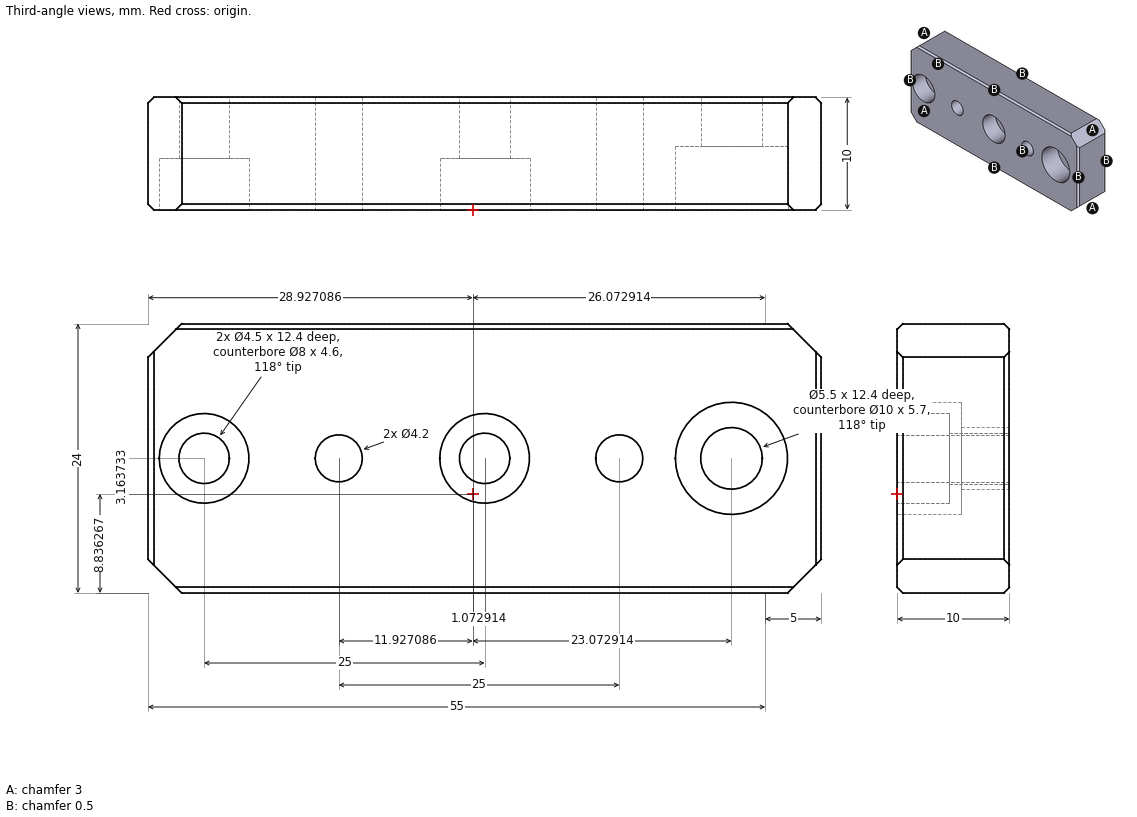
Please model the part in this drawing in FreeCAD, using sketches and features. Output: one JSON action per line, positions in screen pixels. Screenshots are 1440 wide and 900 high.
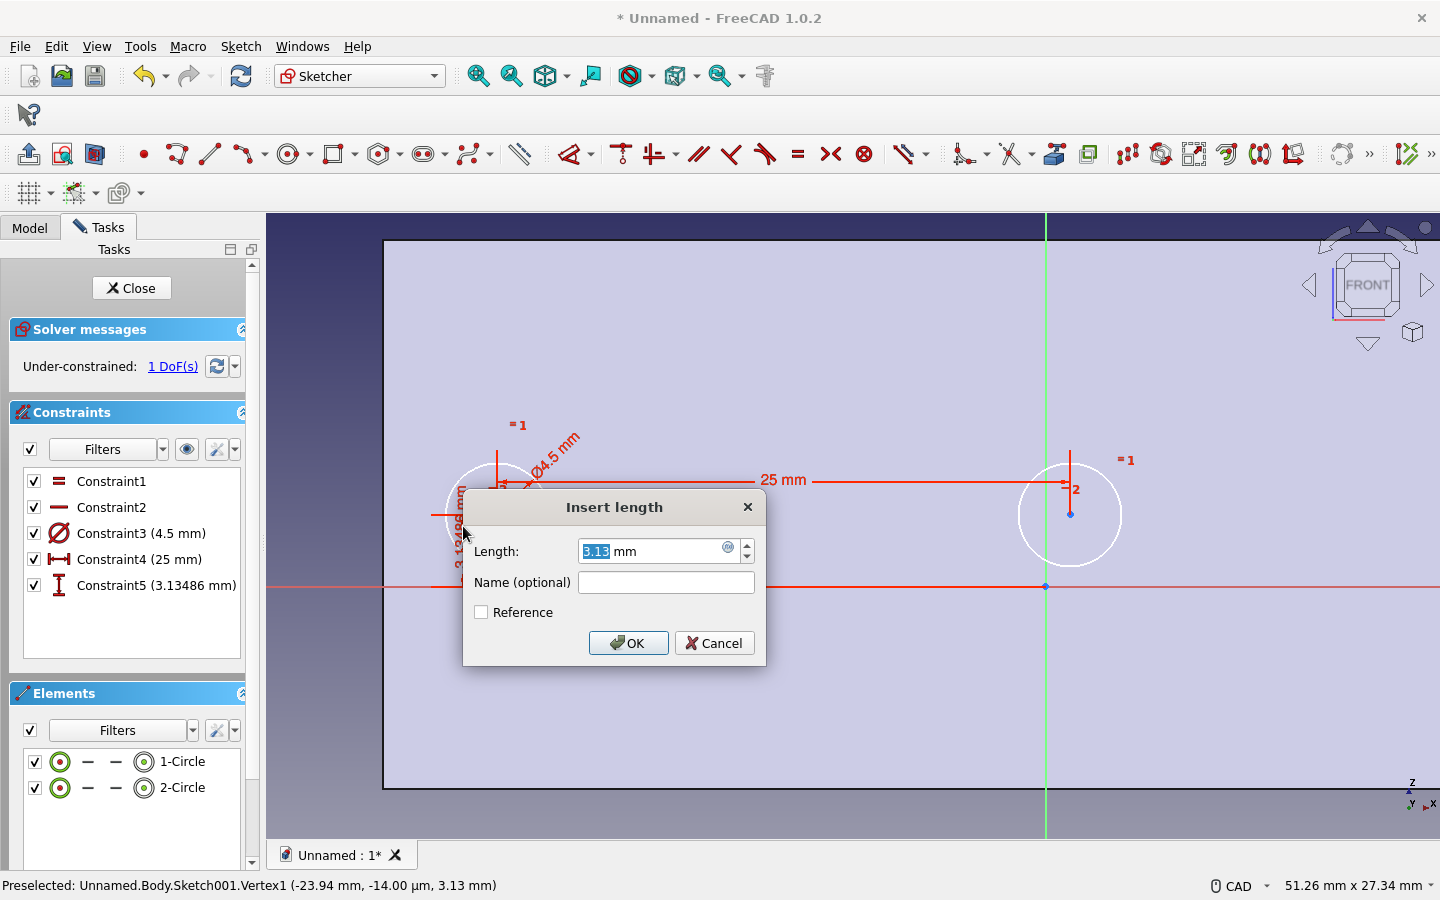
{"action": "type", "text": "3.163733"}
{"action": "key", "text": "Return"}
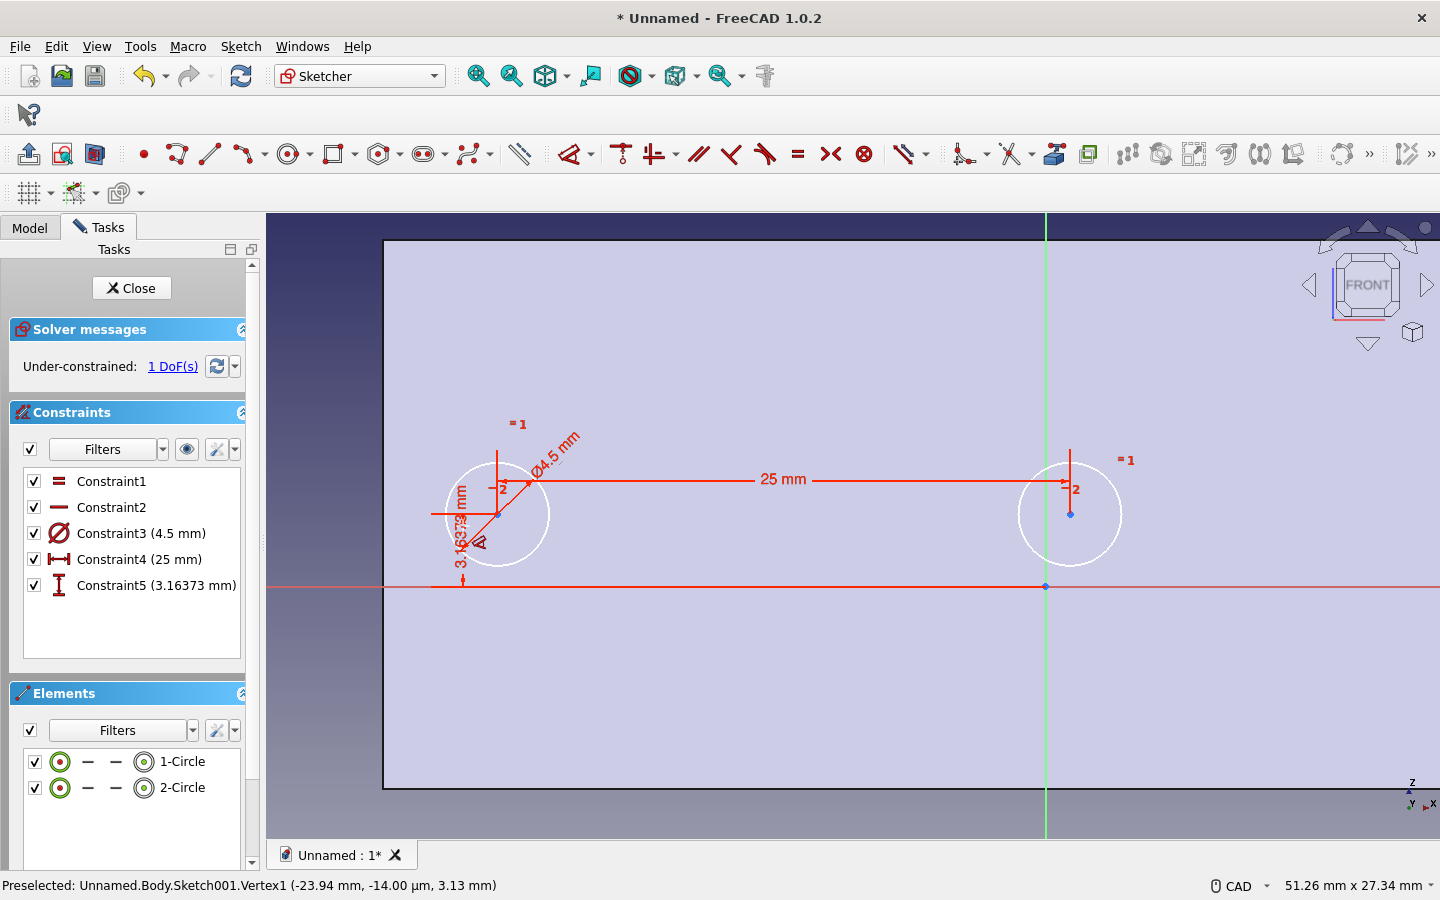
{"action": "scroll", "coordinate": [1070, 514], "scroll_direction": "up", "scroll_amount": 3}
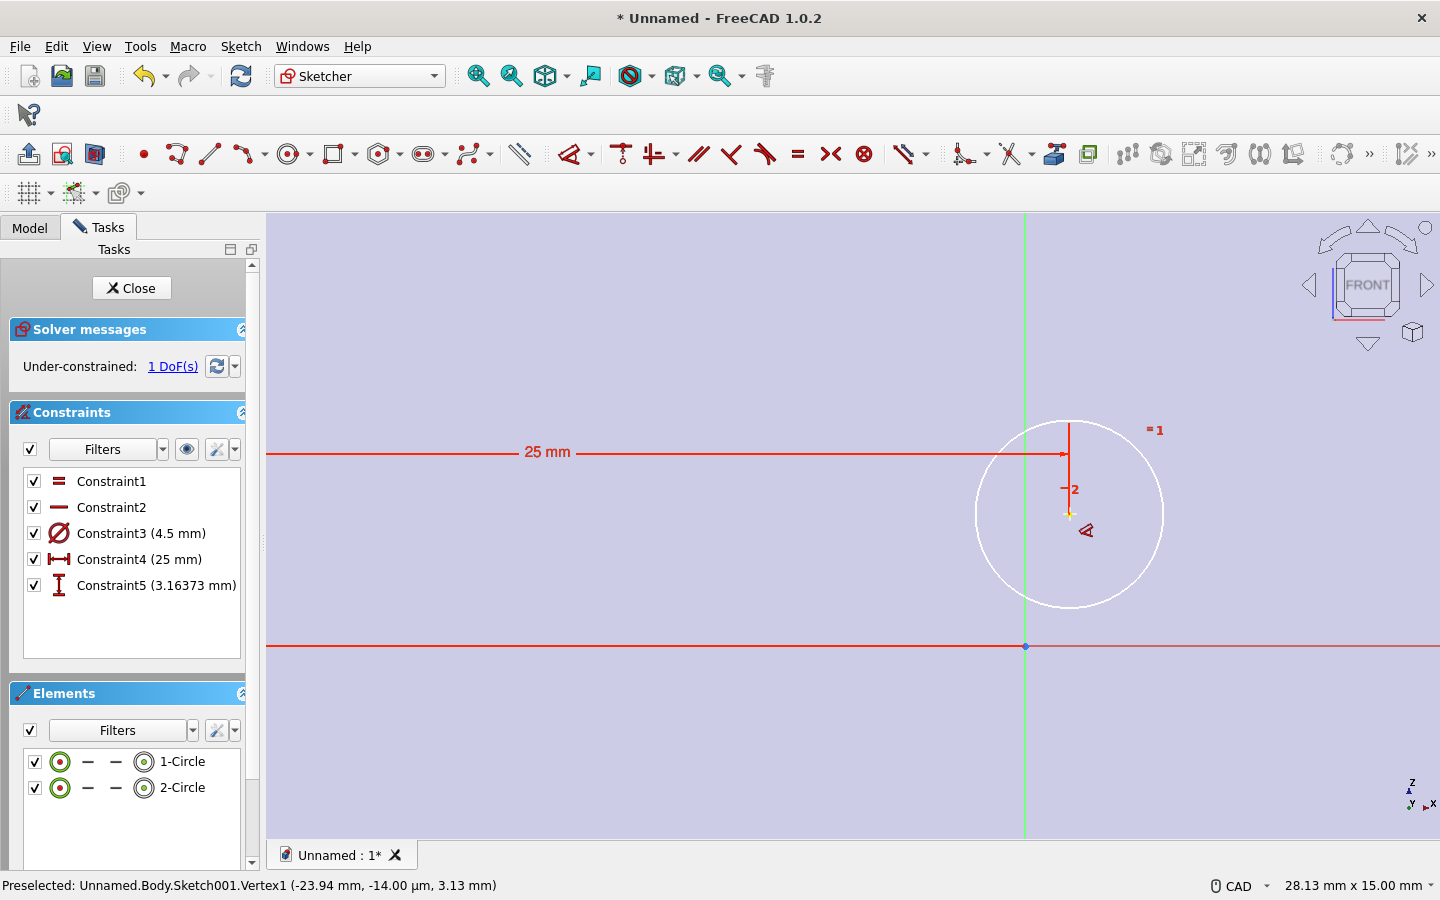
{"action": "left_click", "coordinate": [1069, 514]}
{"action": "left_click", "coordinate": [1047, 680]}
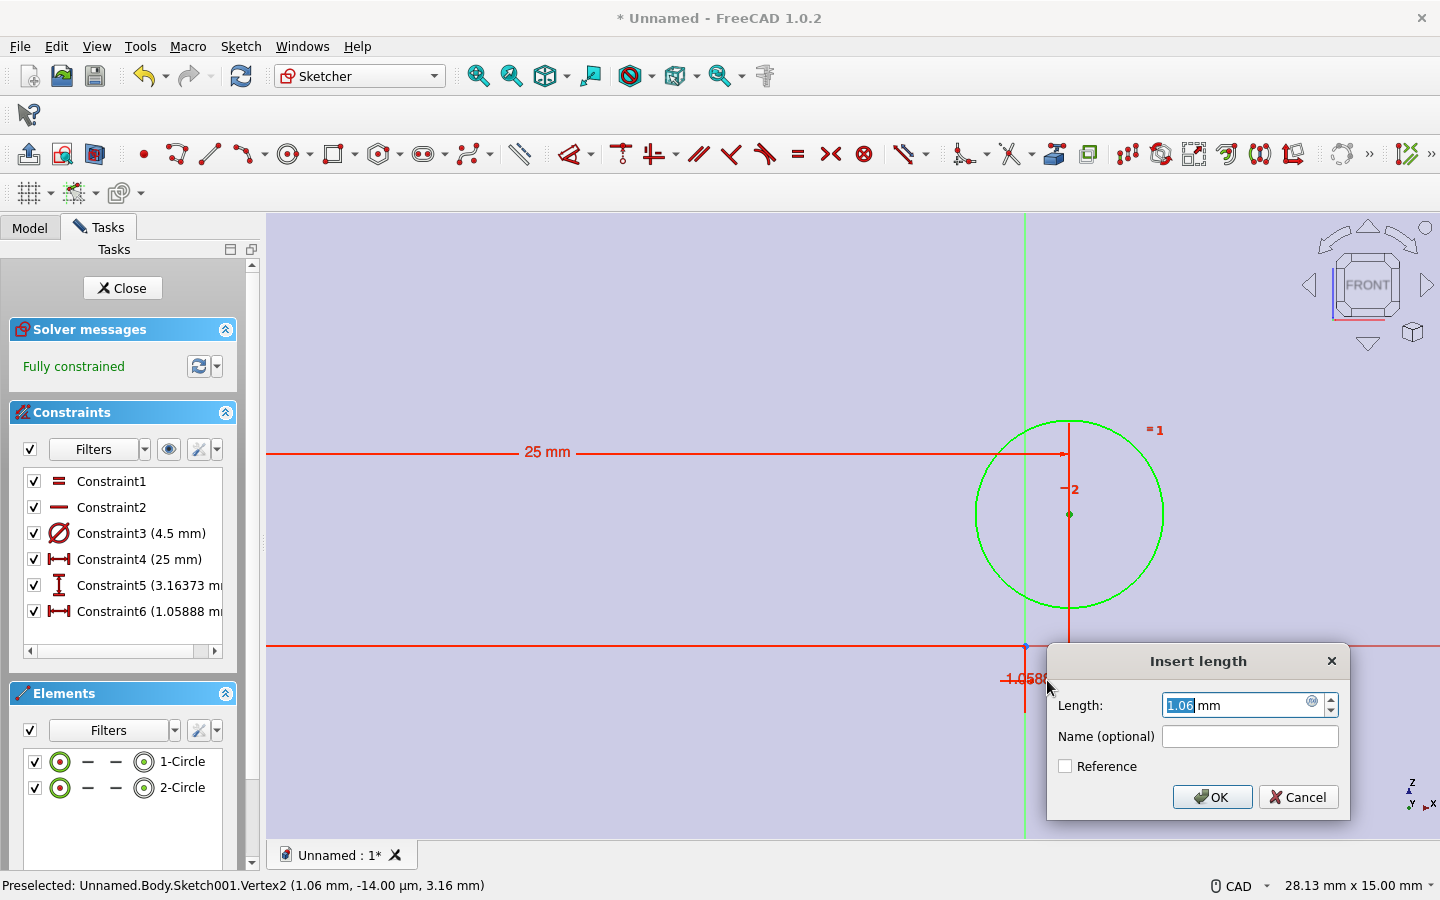
{"action": "type", "text": "1.072914"}
{"action": "key", "text": "Return"}
{"action": "key", "text": "Escape"}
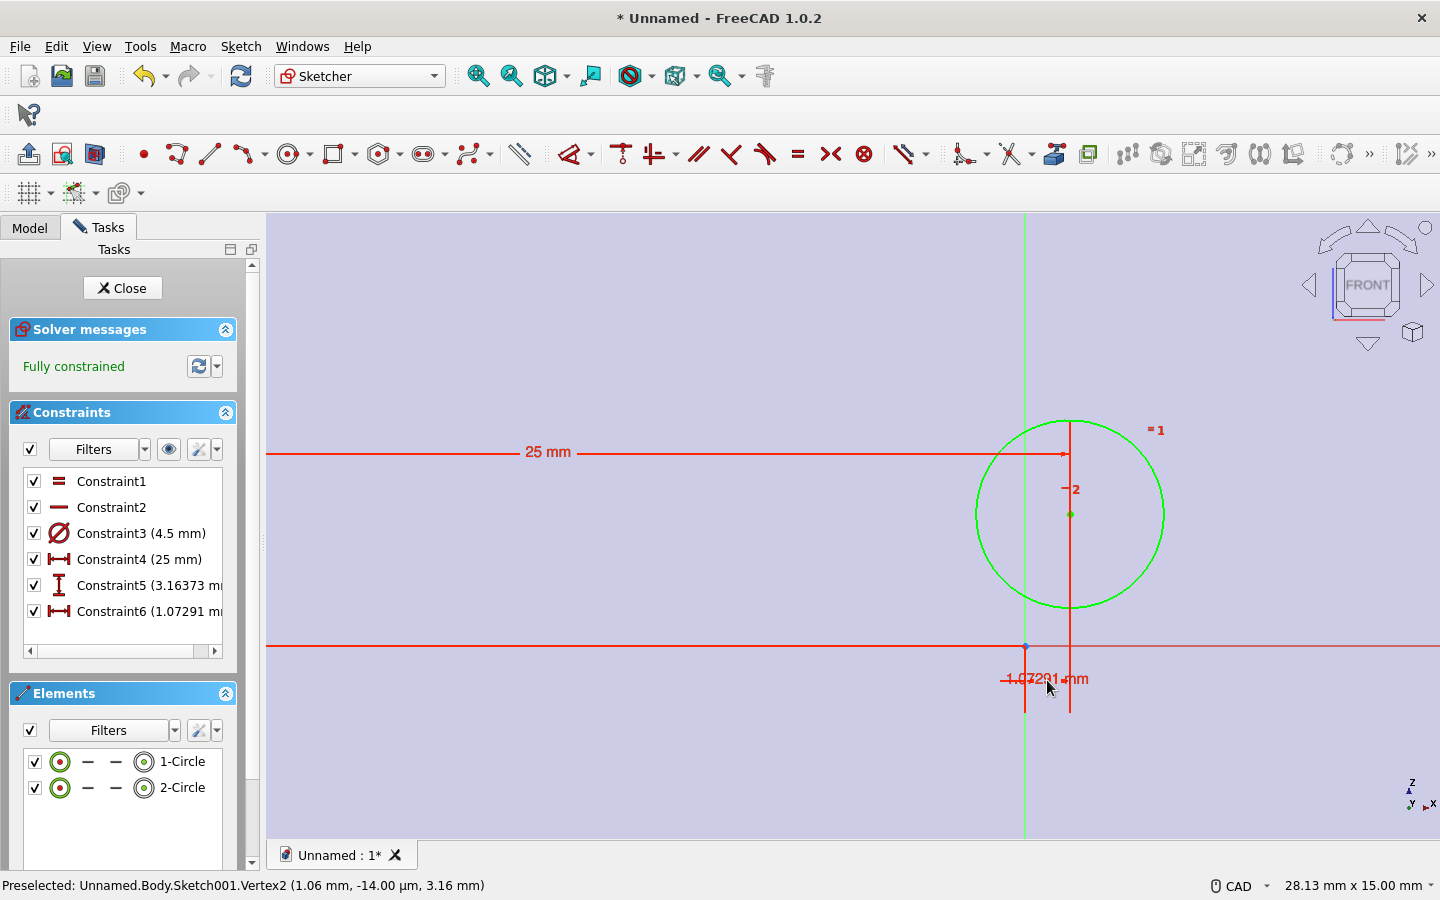
{"action": "left_click", "coordinate": [123, 288]}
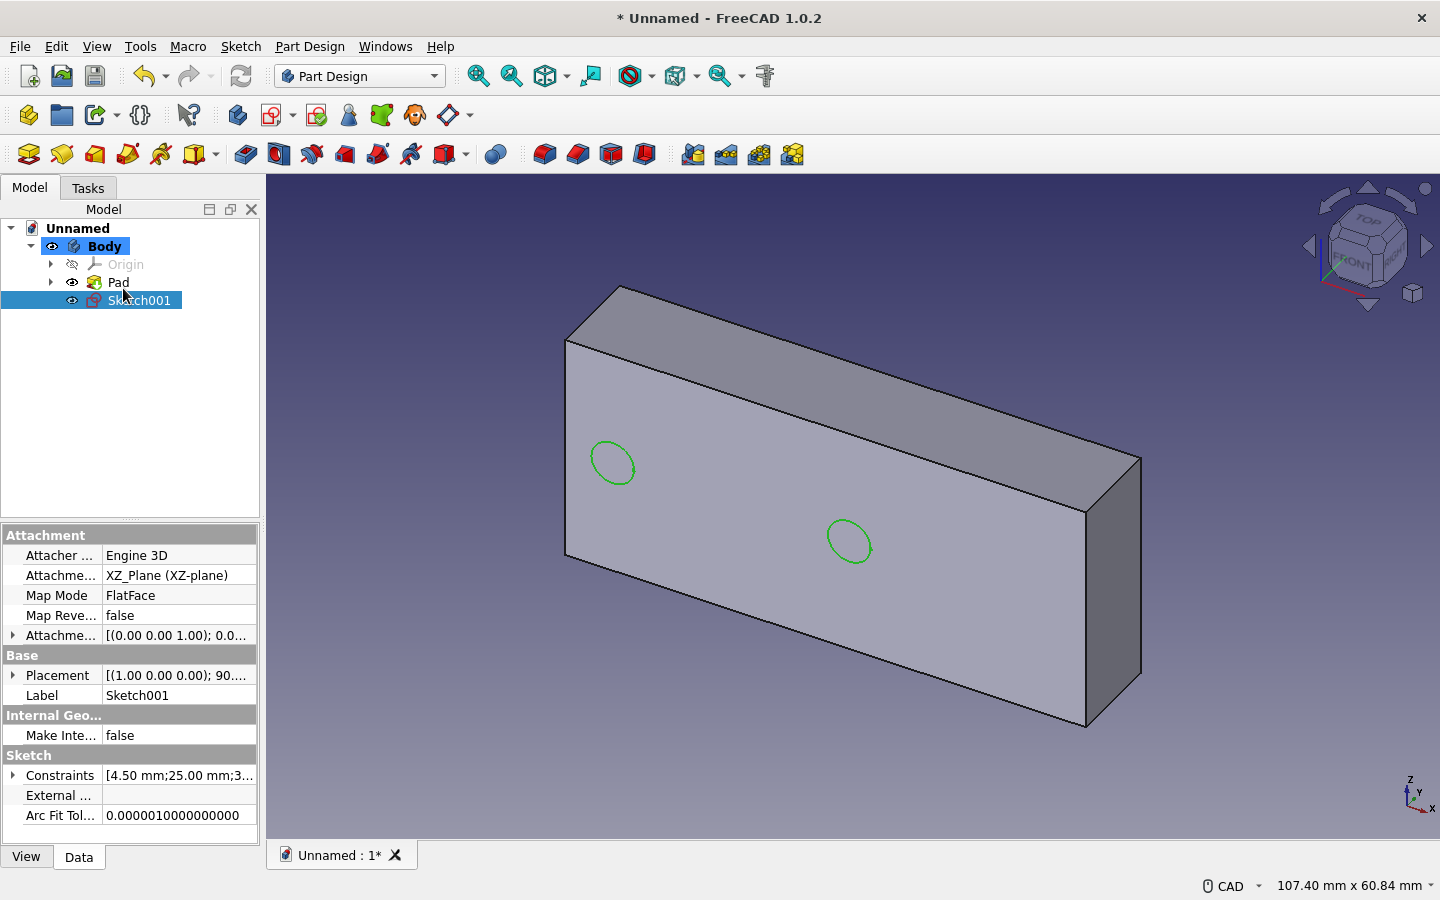
{"action": "left_click", "coordinate": [279, 154]}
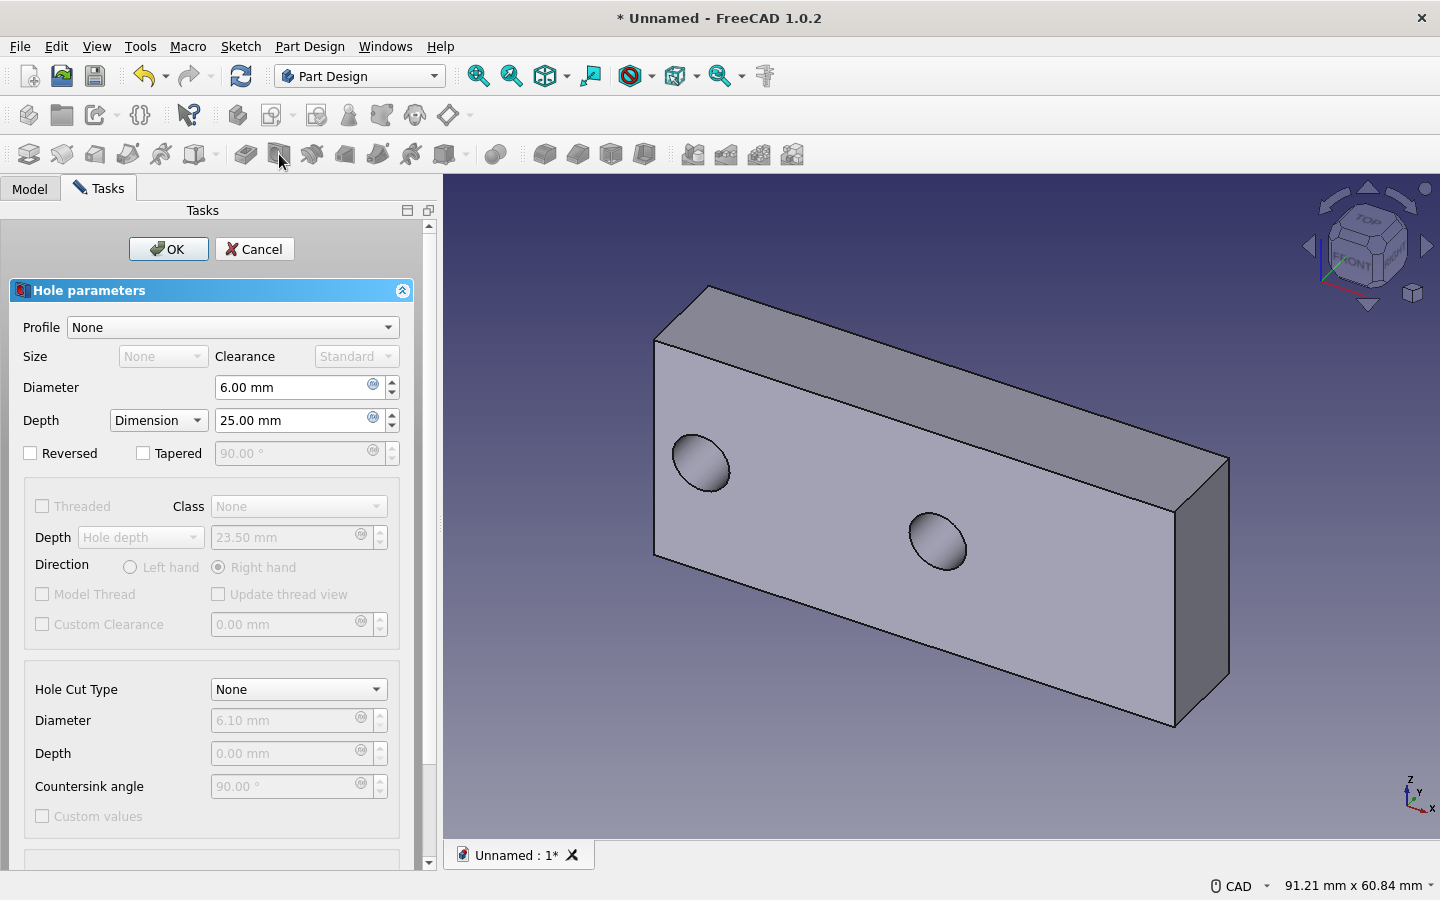
{"action": "triple_click", "coordinate": [300, 388]}